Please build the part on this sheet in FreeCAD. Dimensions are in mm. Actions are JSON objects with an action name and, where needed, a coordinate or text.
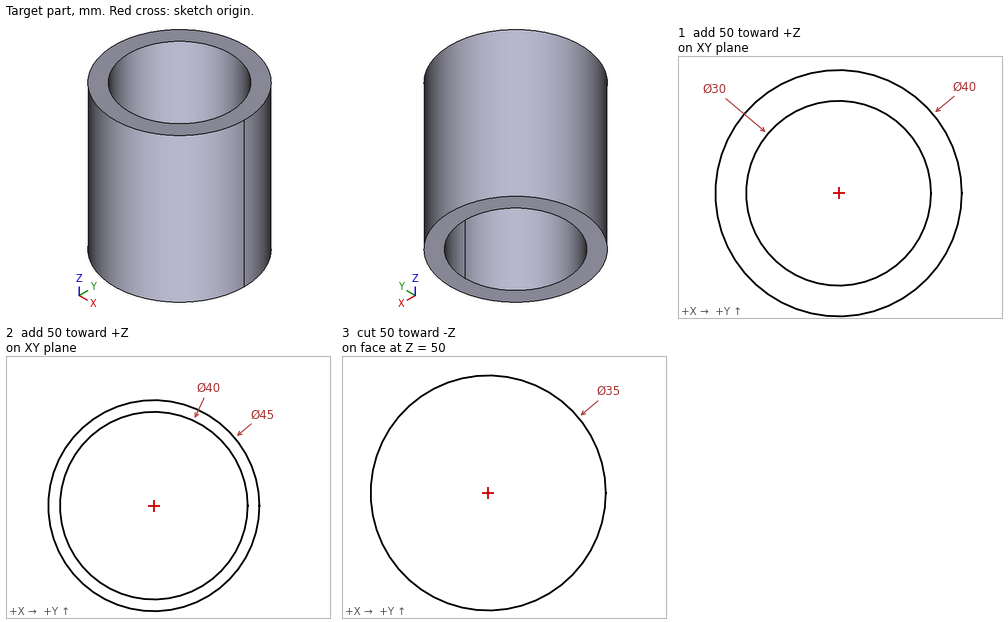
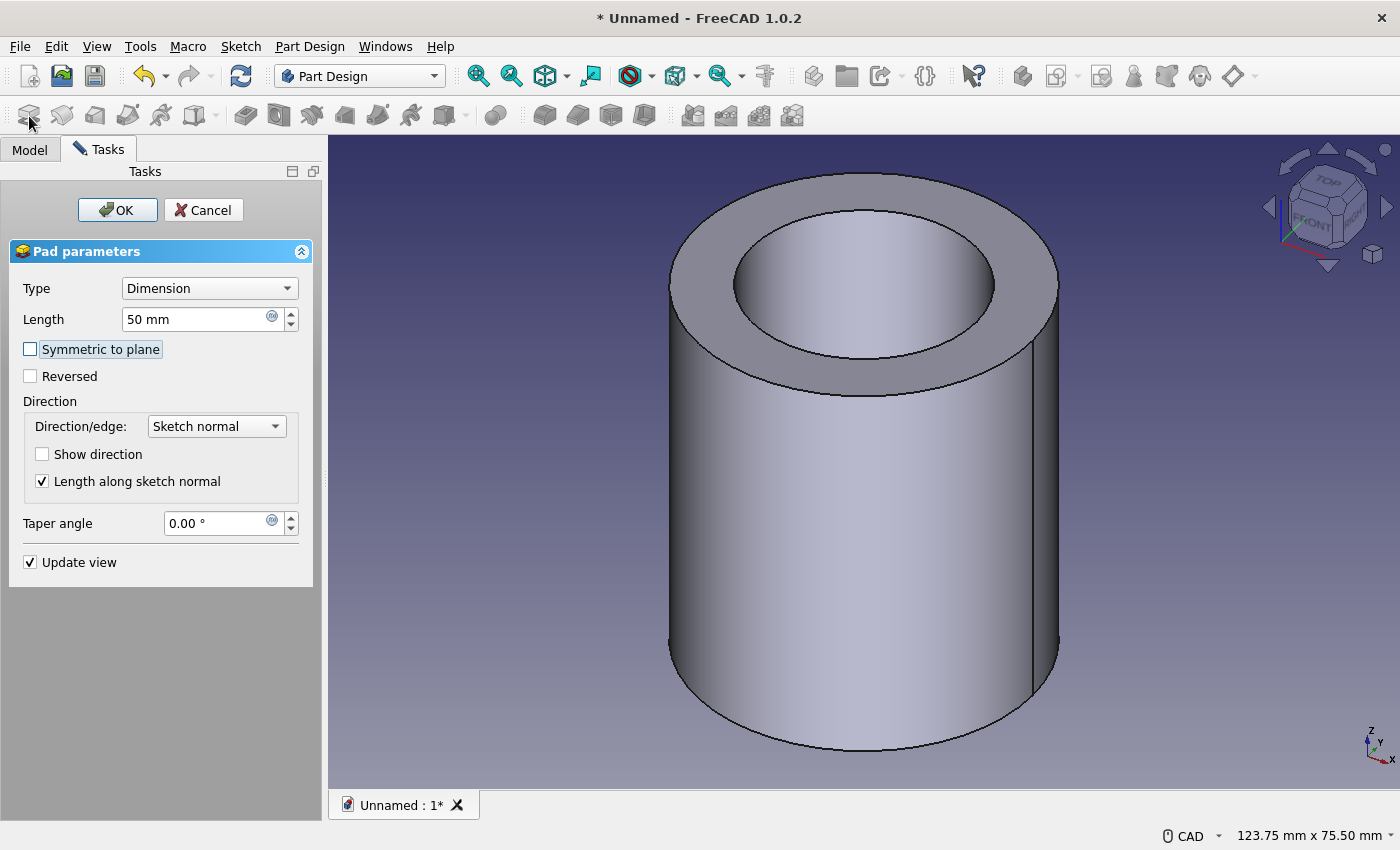
{"action": "left_click", "coordinate": [118, 210]}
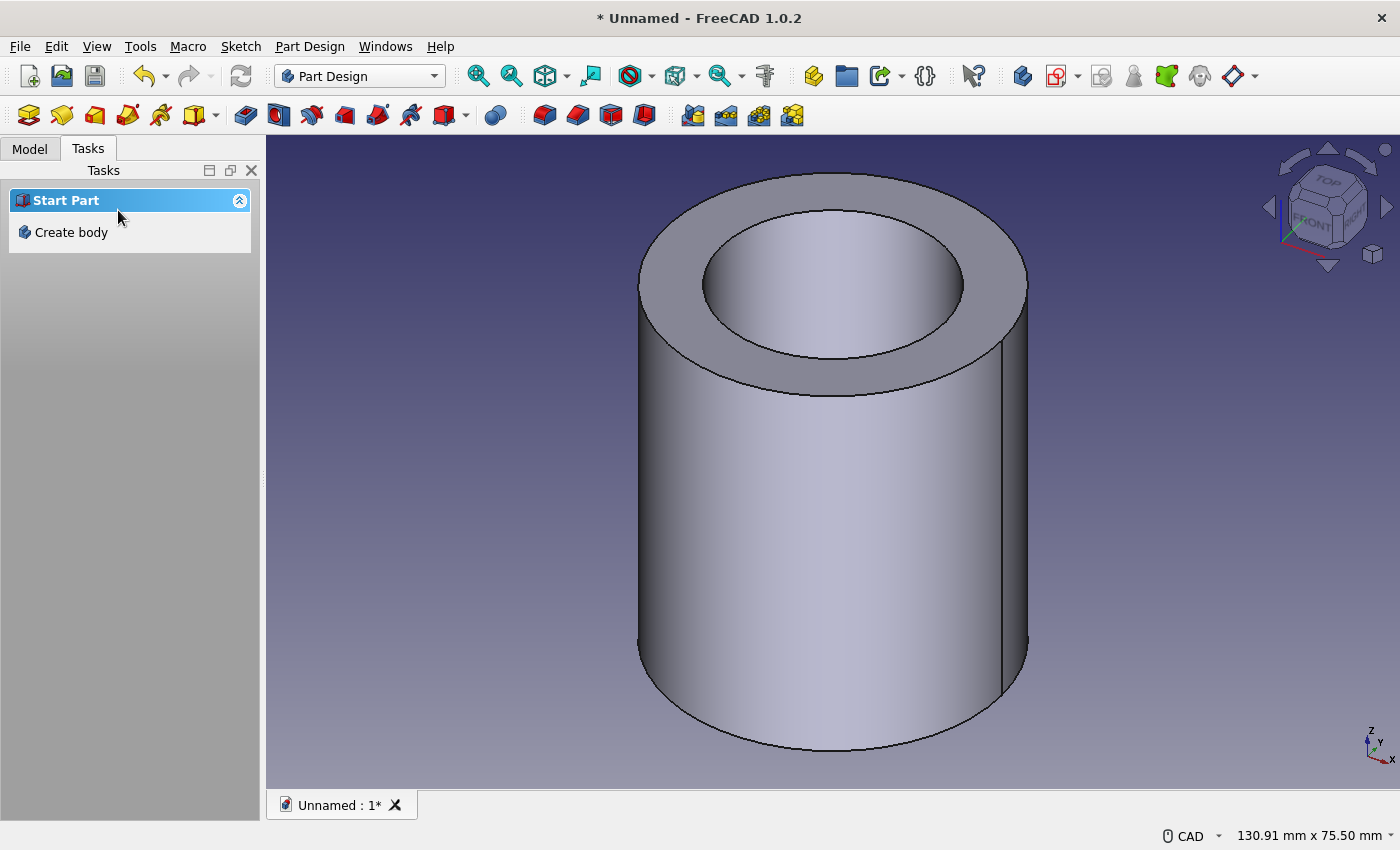
{"action": "left_click", "coordinate": [479, 76]}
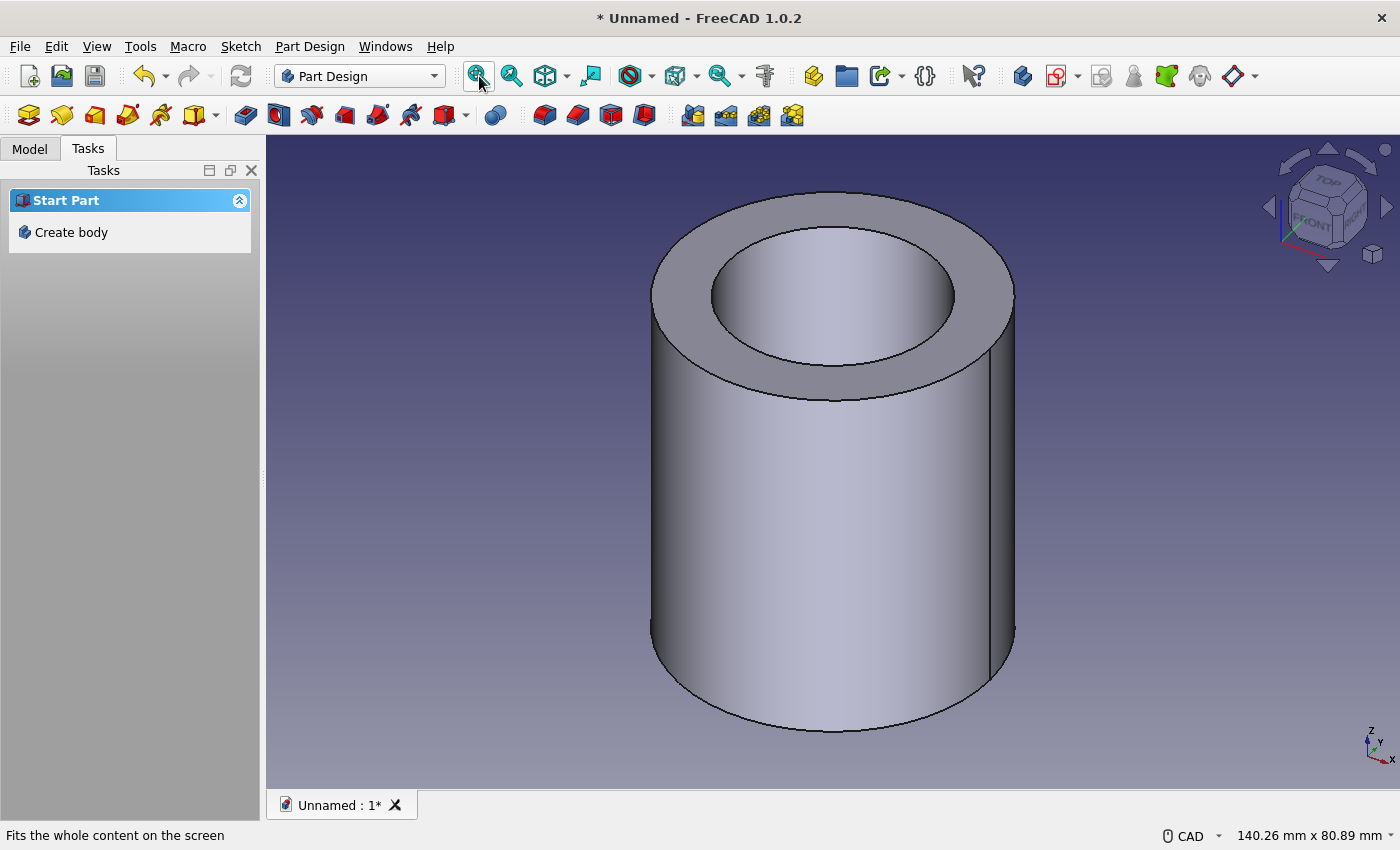
{"action": "left_click", "coordinate": [968, 340]}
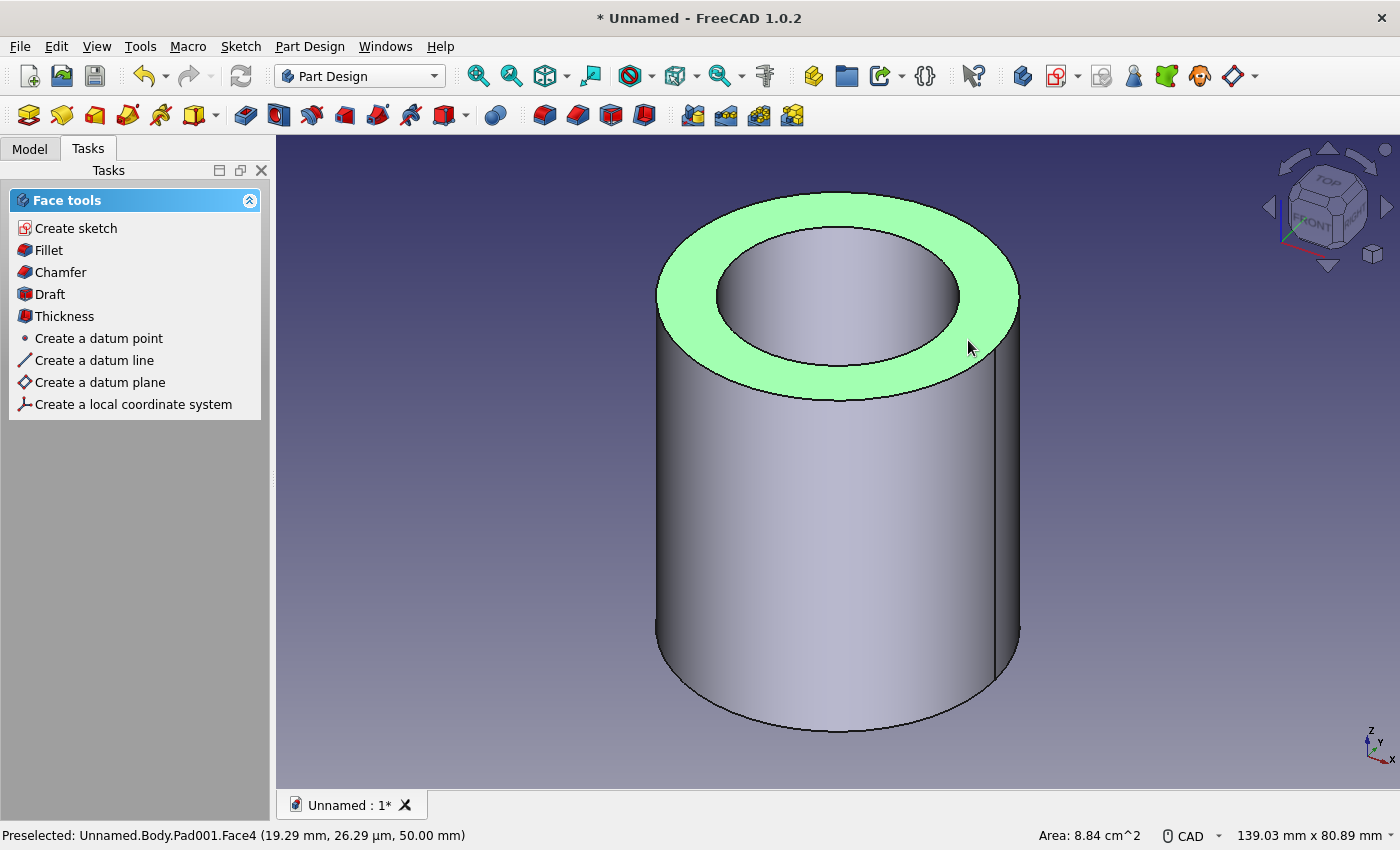
{"action": "left_click", "coordinate": [1056, 76]}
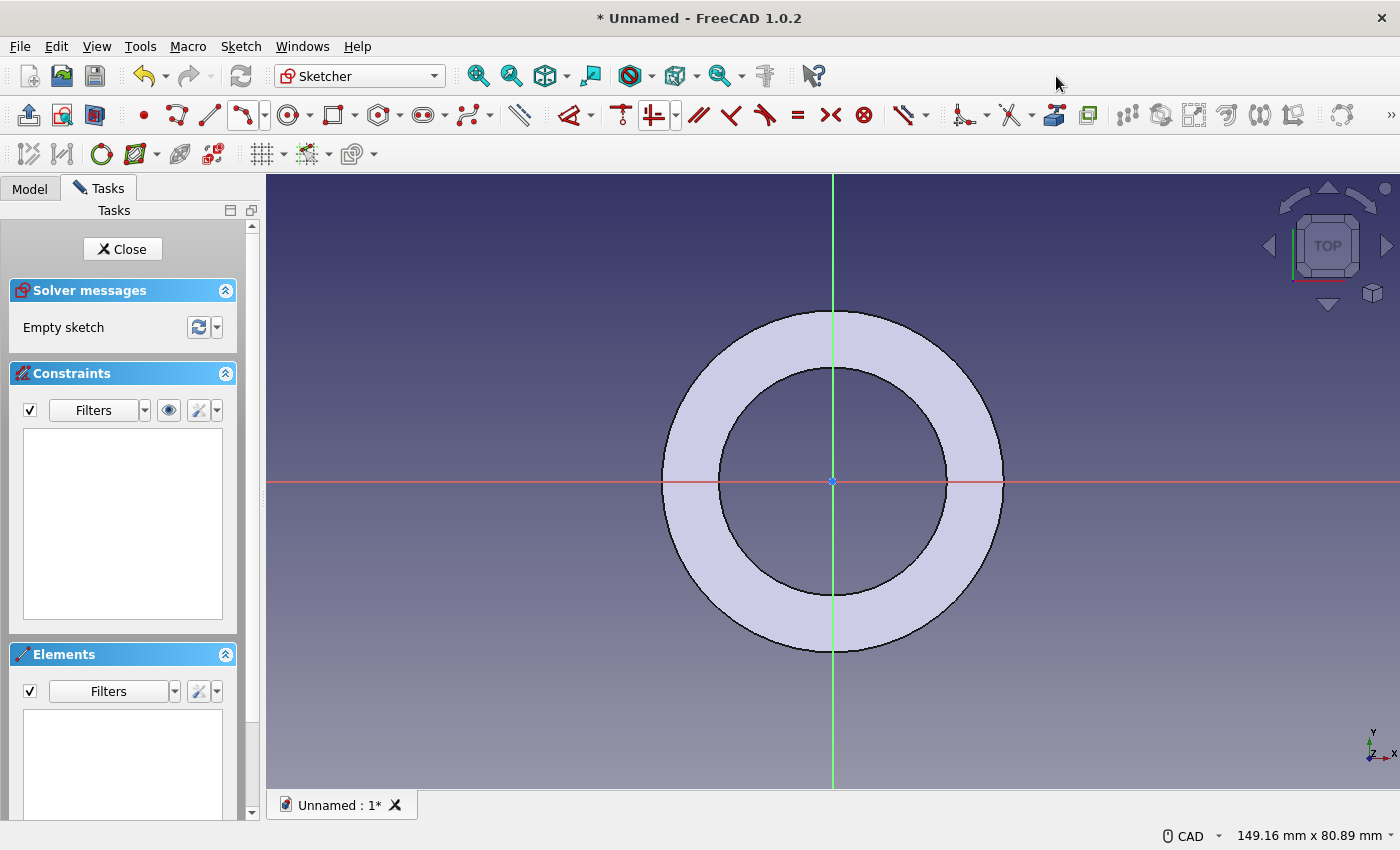
{"action": "scroll", "coordinate": [972, 482], "scroll_direction": "up", "scroll_amount": 2}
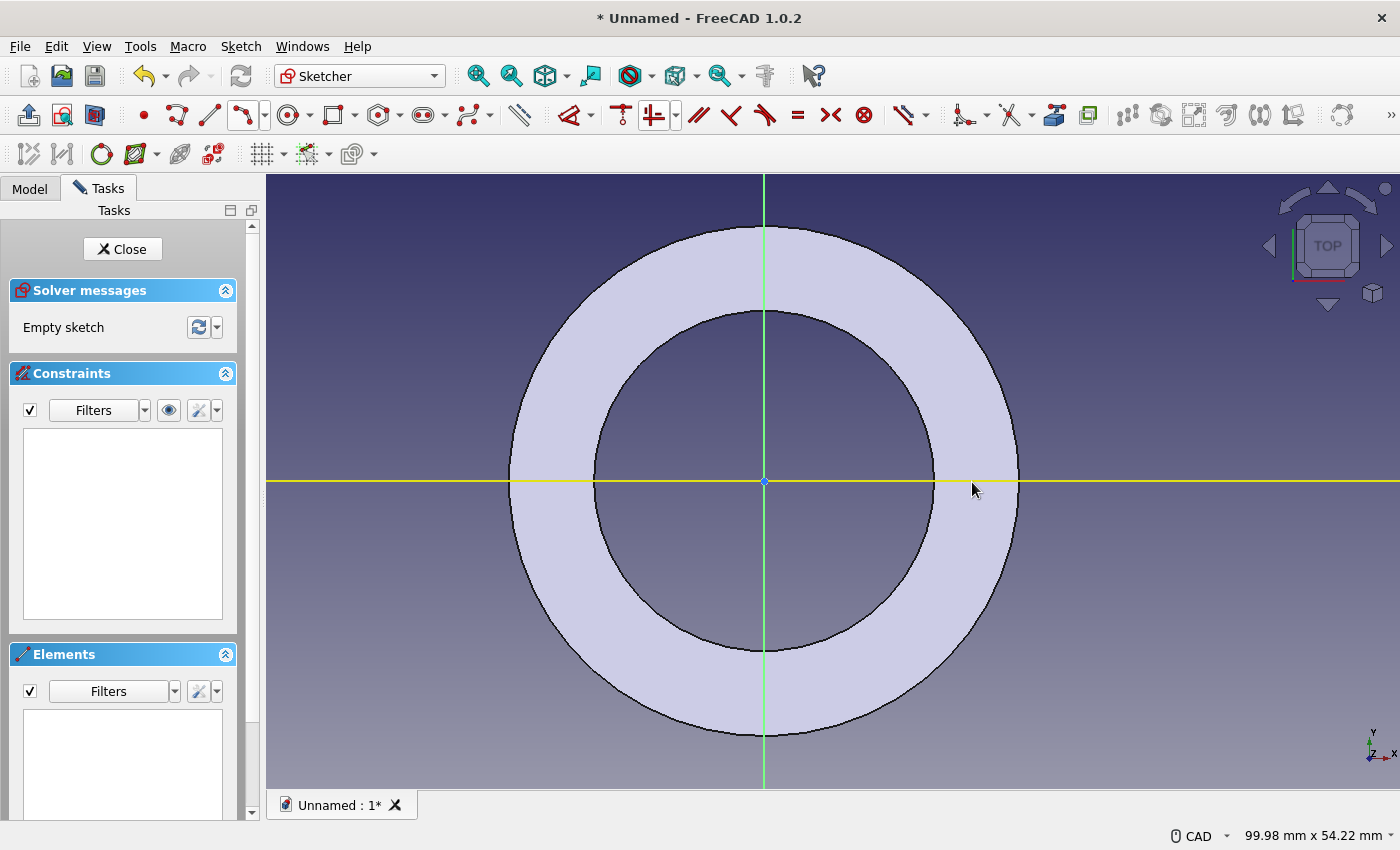
{"action": "left_click", "coordinate": [288, 116]}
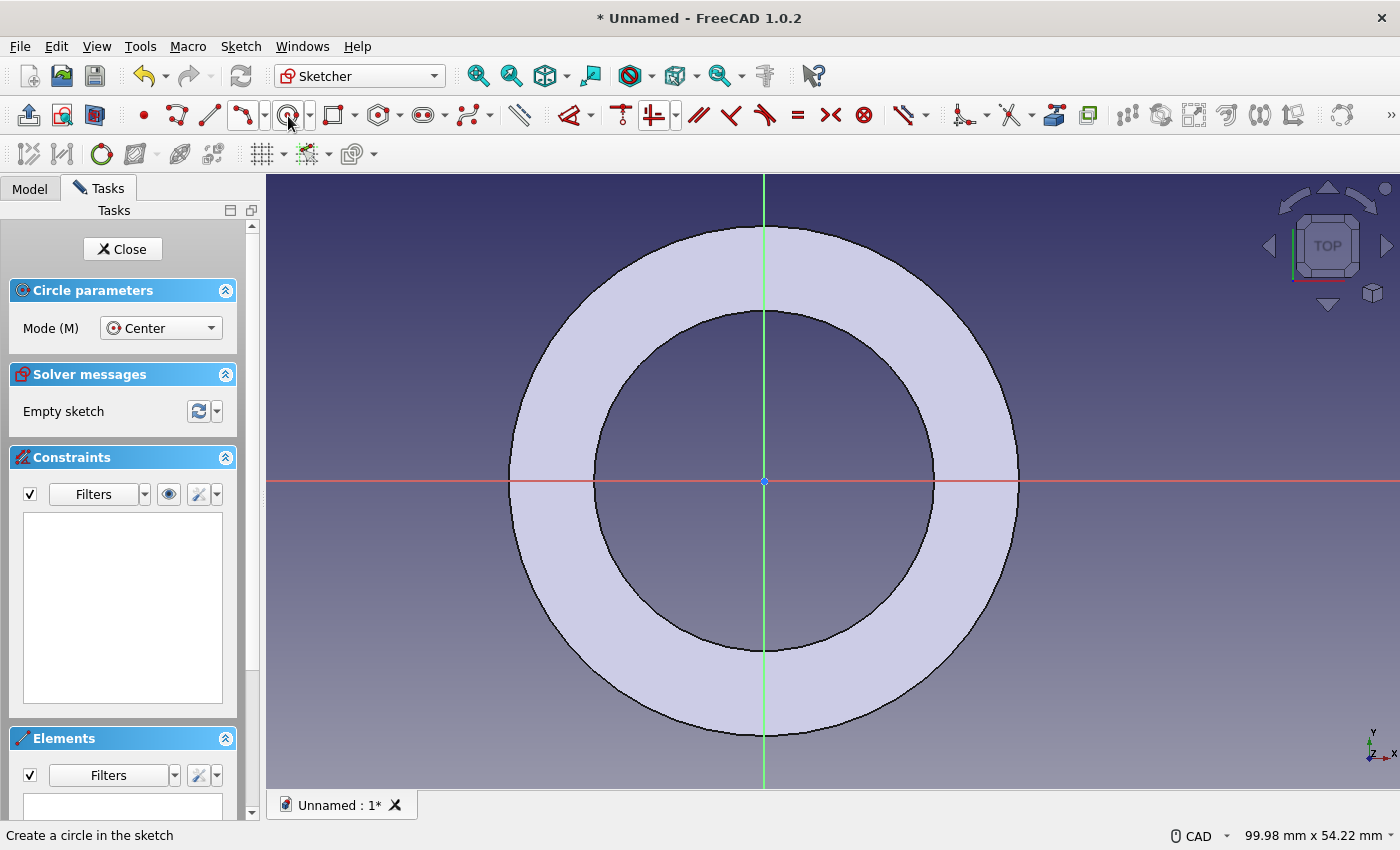
{"action": "left_click", "coordinate": [764, 481]}
{"action": "mouse_move", "coordinate": [904, 341]}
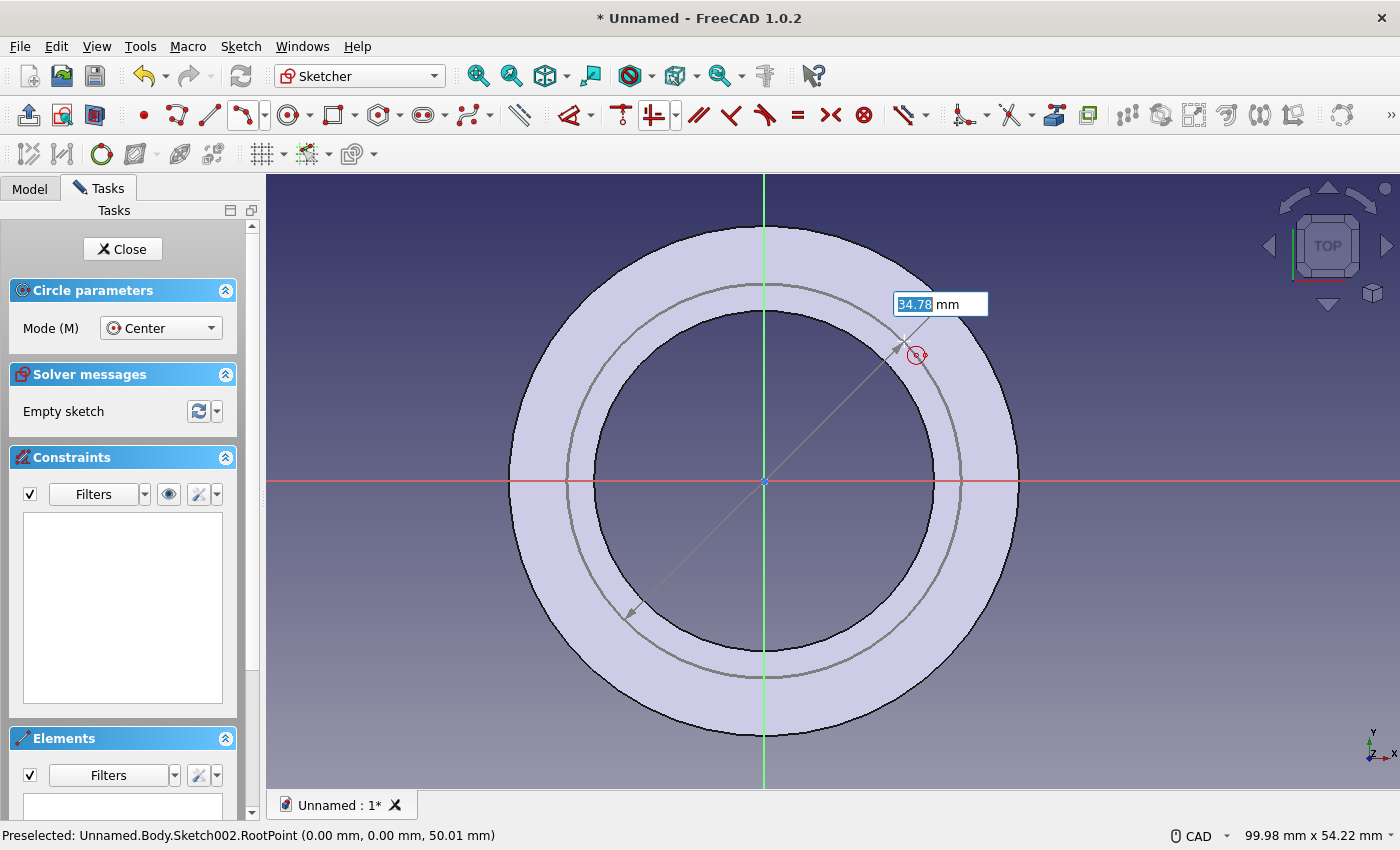
{"action": "type", "text": "35"}
{"action": "key", "text": "Return"}
{"action": "key", "text": "Escape"}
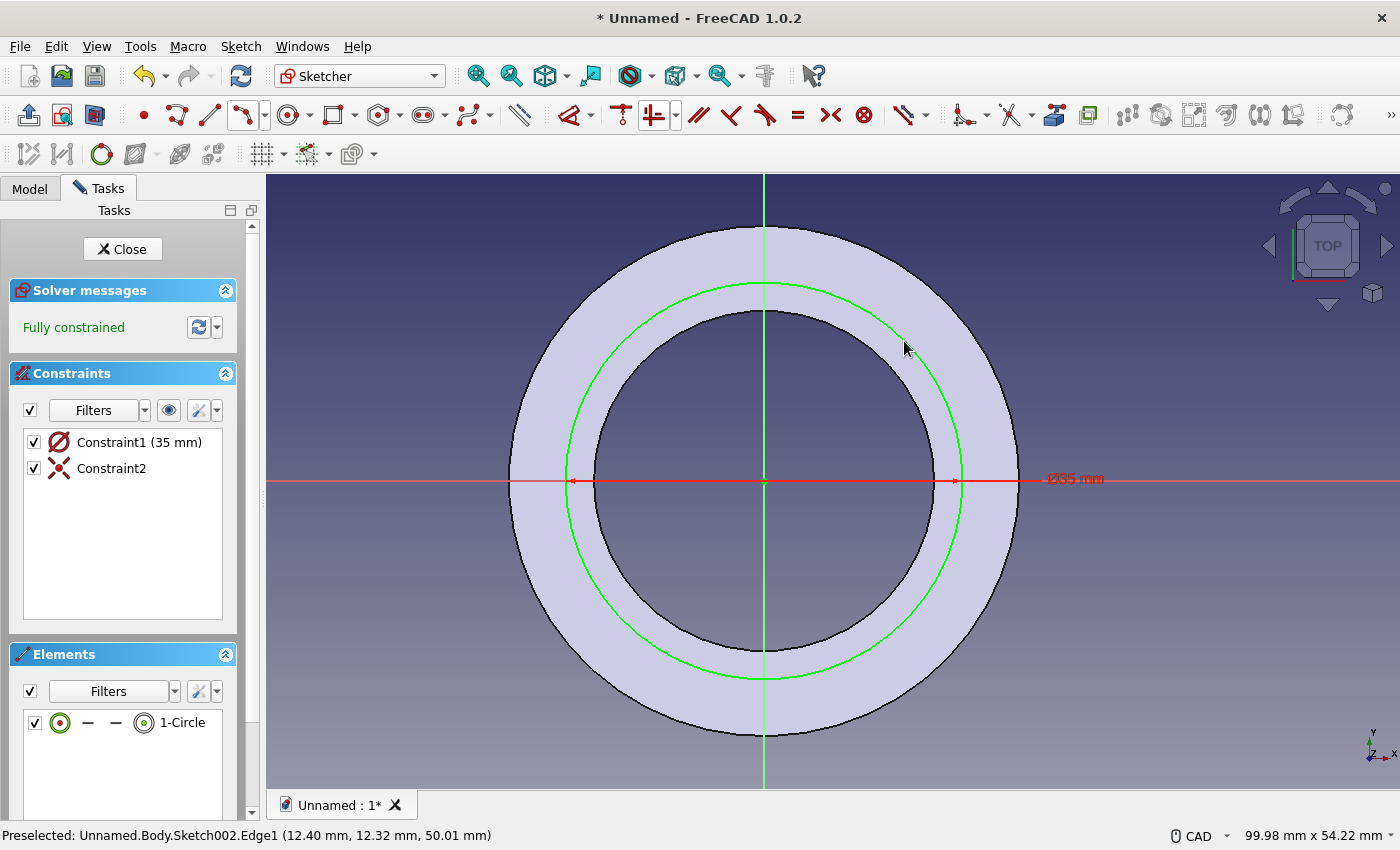
{"action": "left_click", "coordinate": [123, 249]}